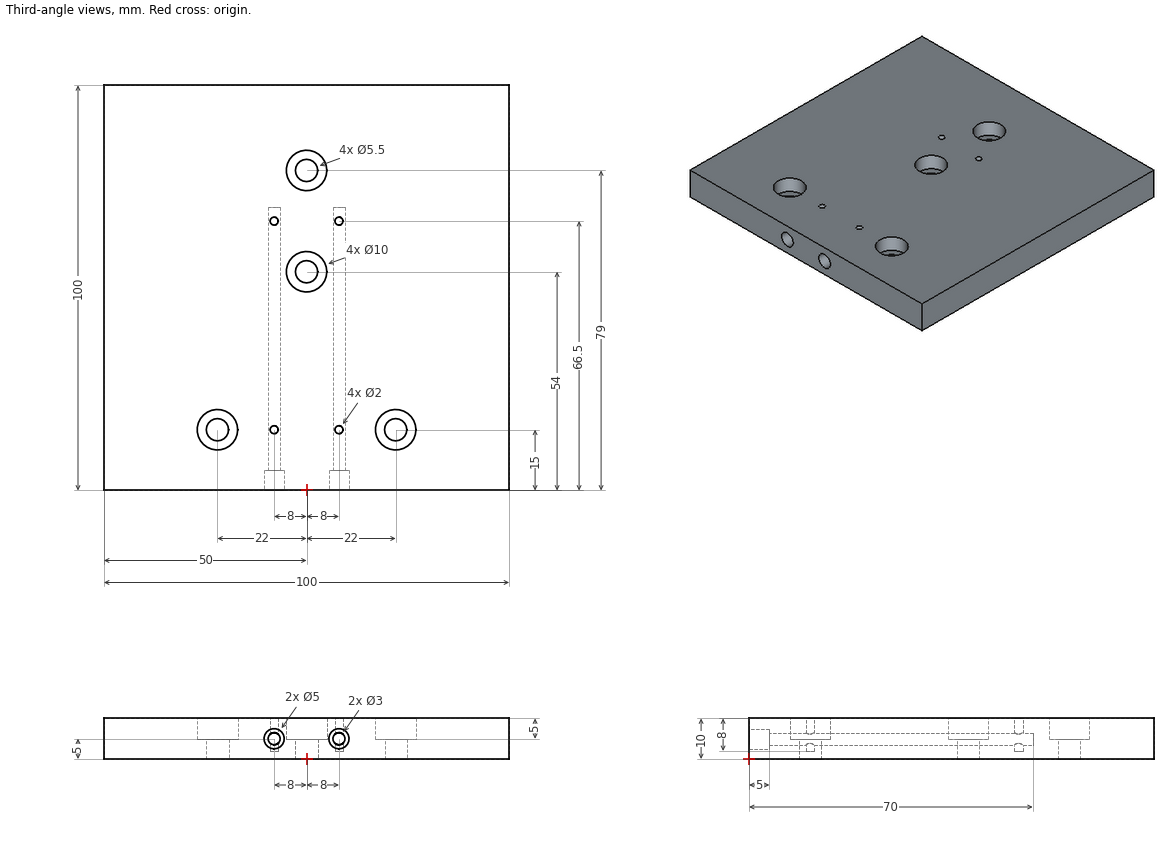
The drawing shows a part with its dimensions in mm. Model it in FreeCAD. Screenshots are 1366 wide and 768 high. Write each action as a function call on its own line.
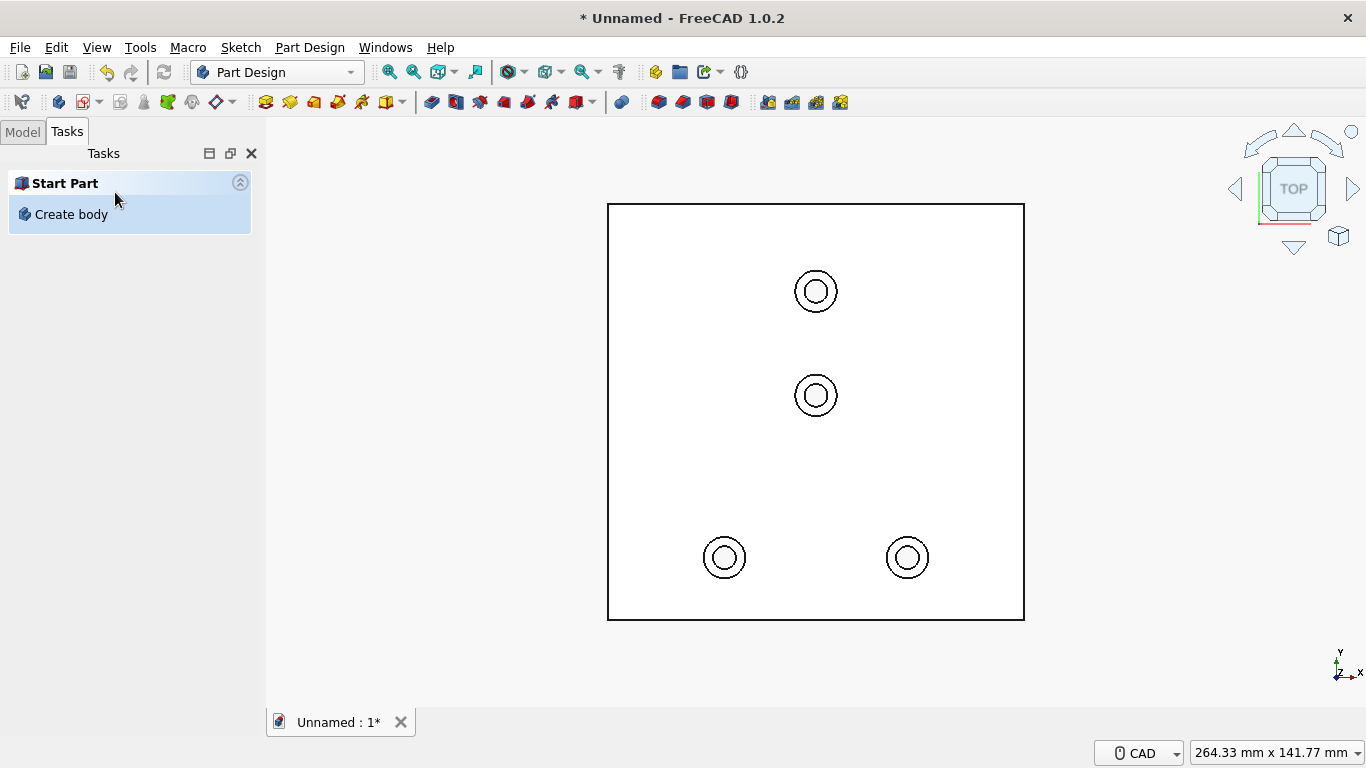
click(935, 352)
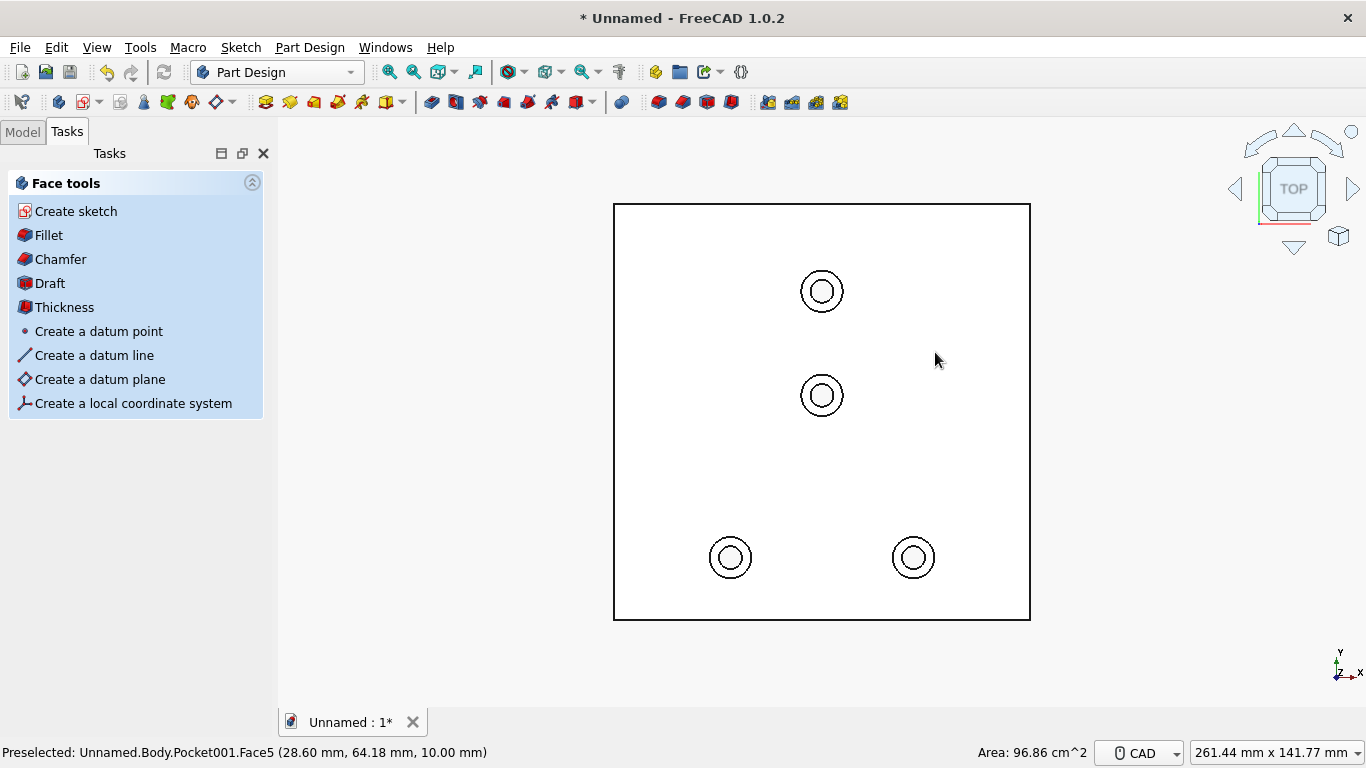
click(84, 102)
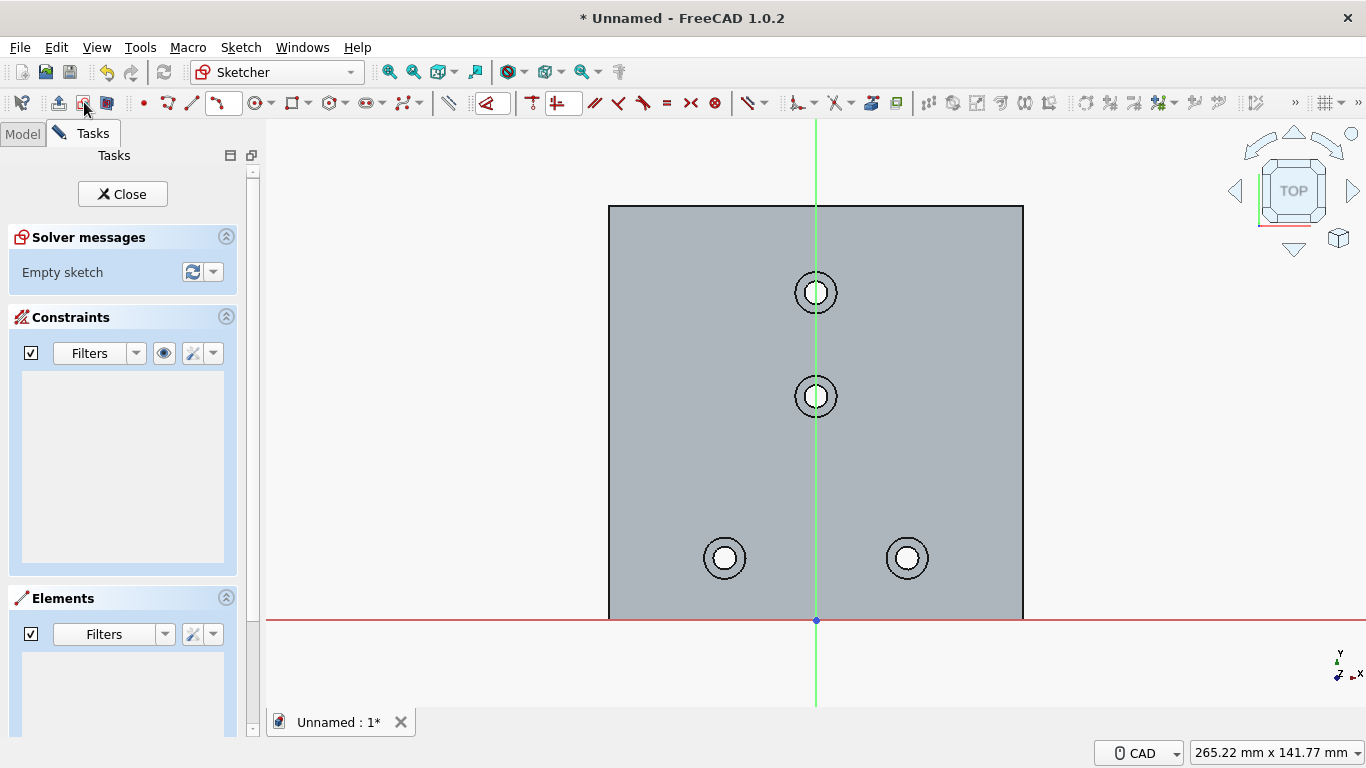
click(256, 104)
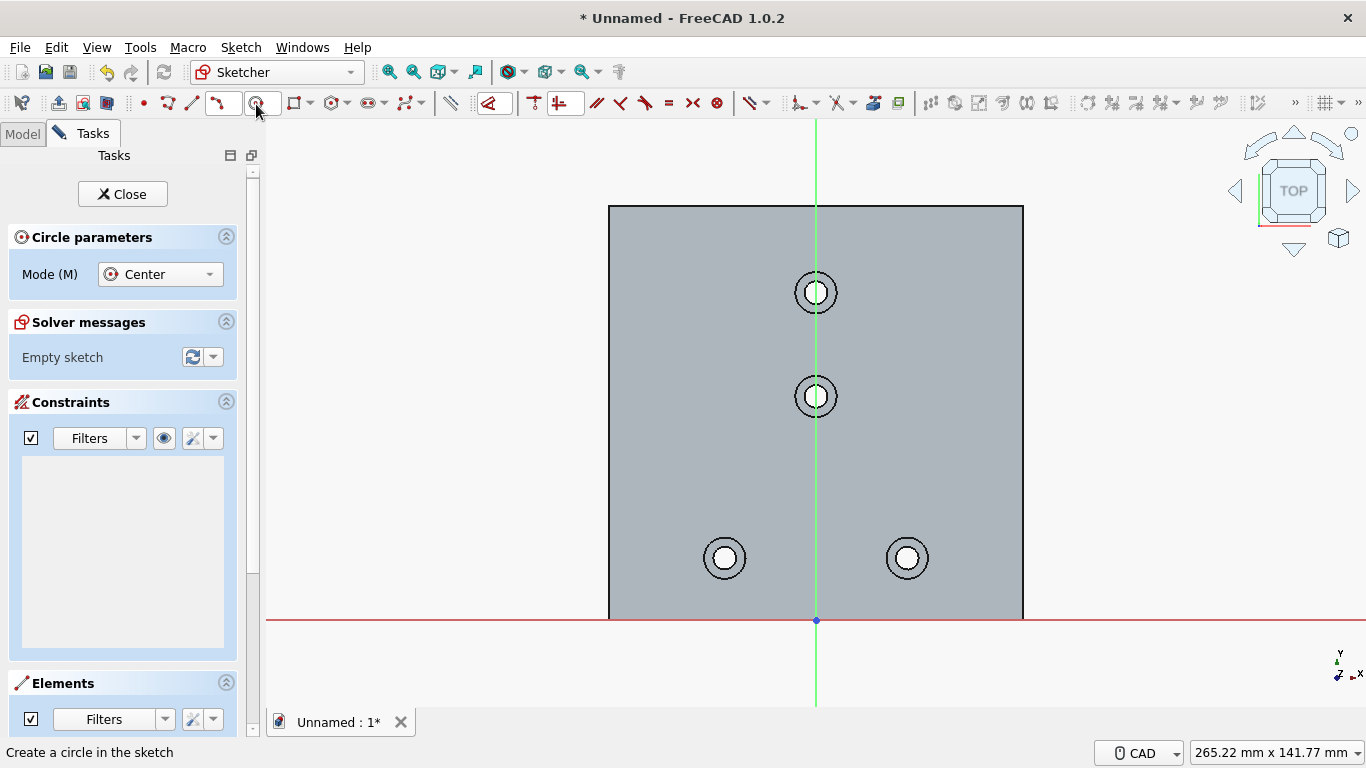
scroll(849, 558, up, 9)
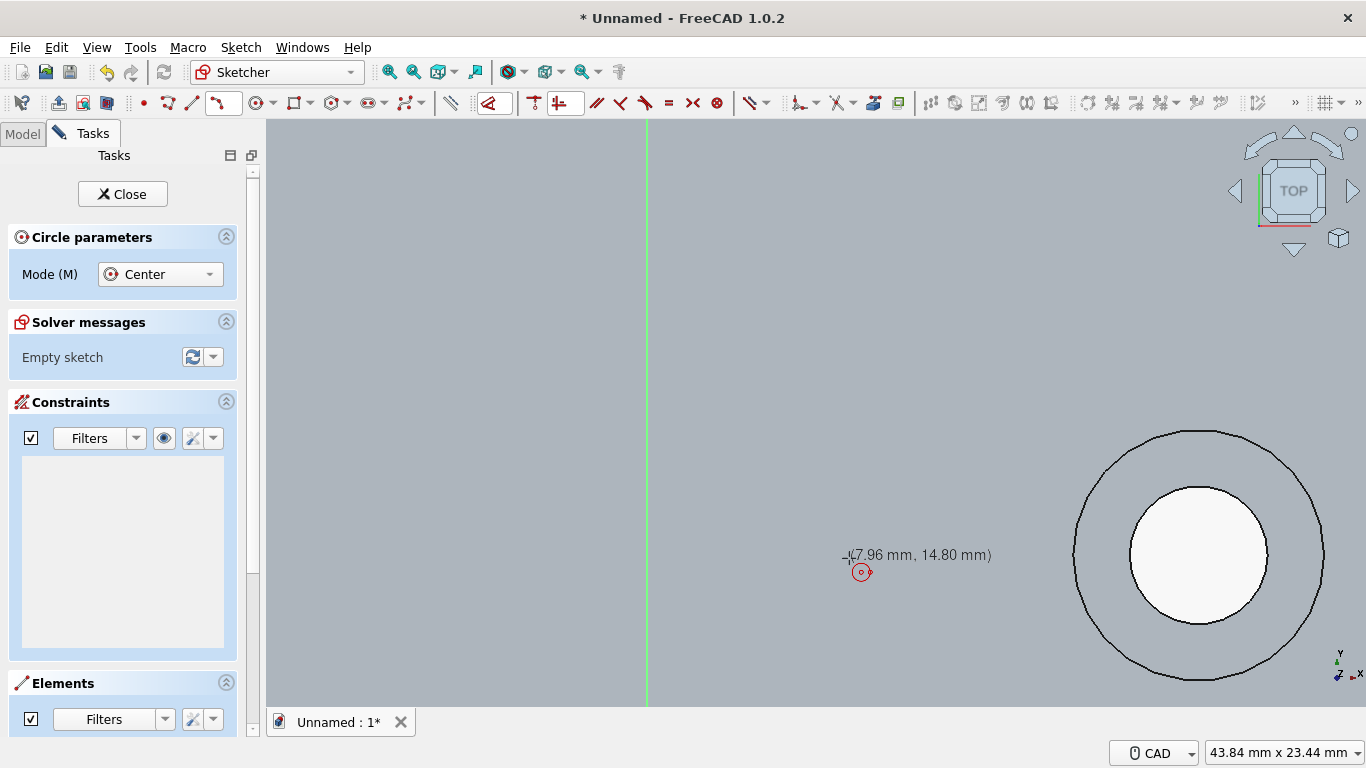
scroll(773, 496, down, 8)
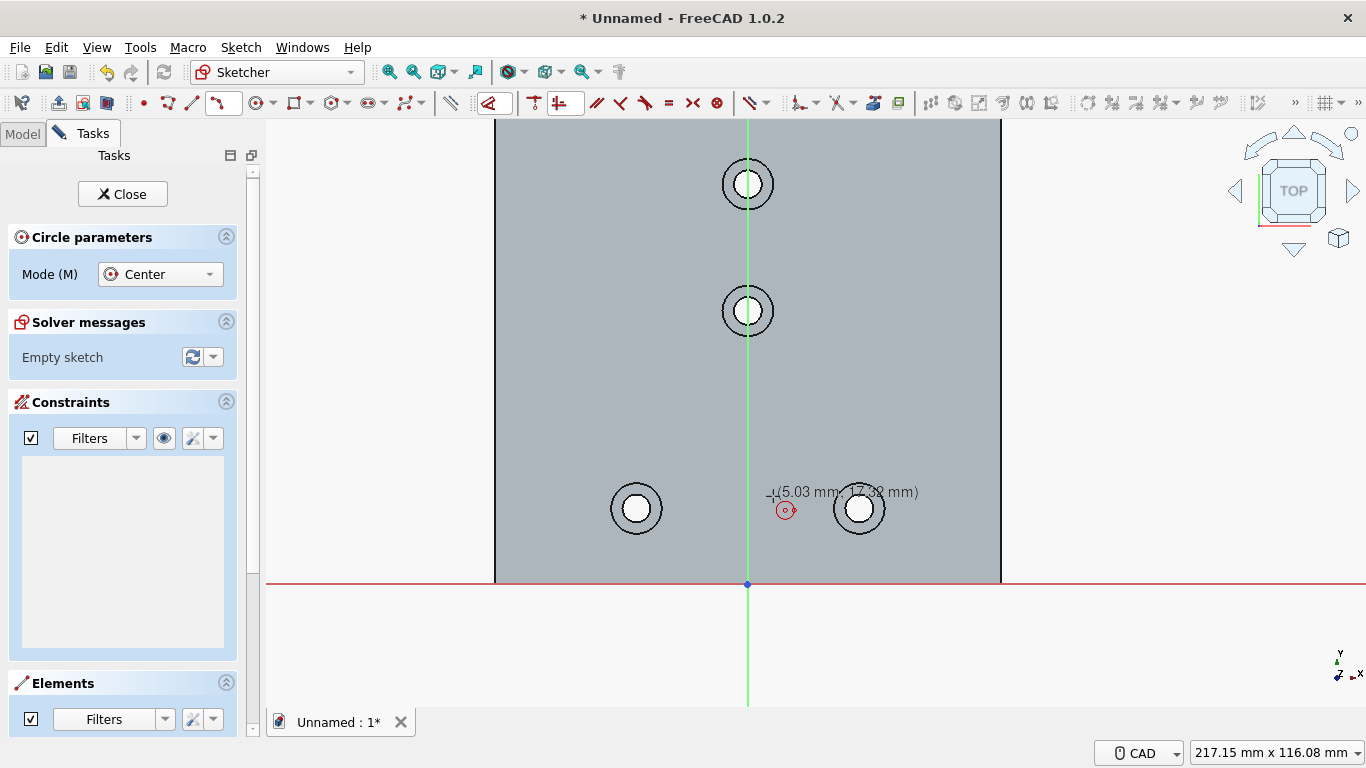
click(788, 508)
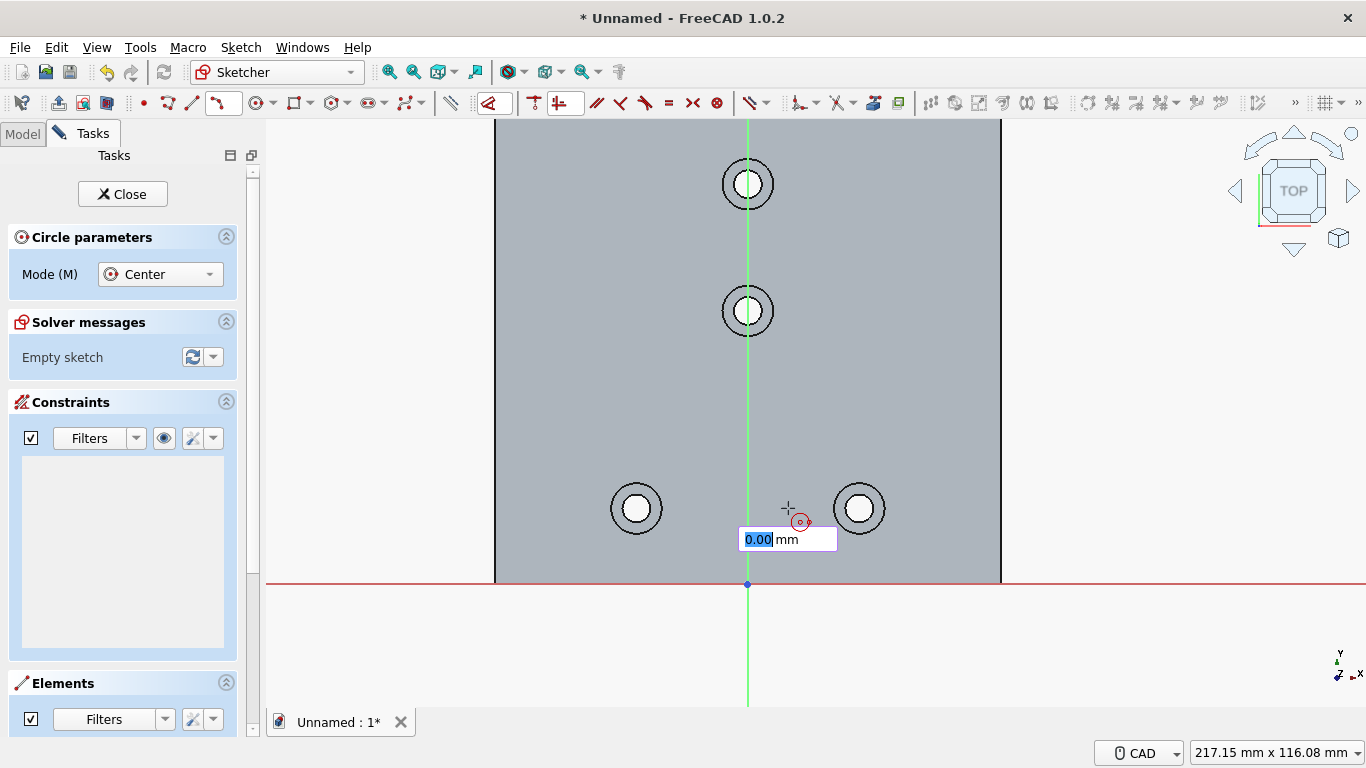
scroll(792, 505, up, 6)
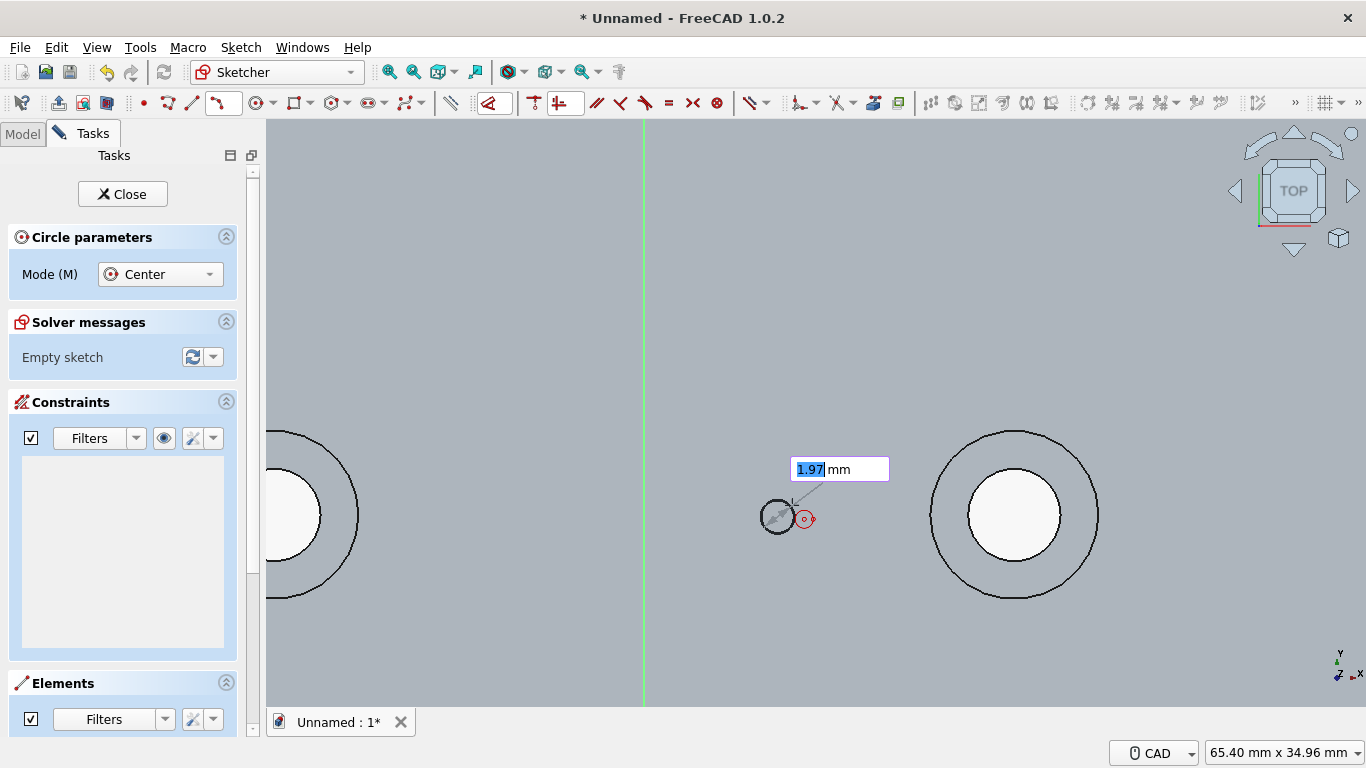
click(791, 503)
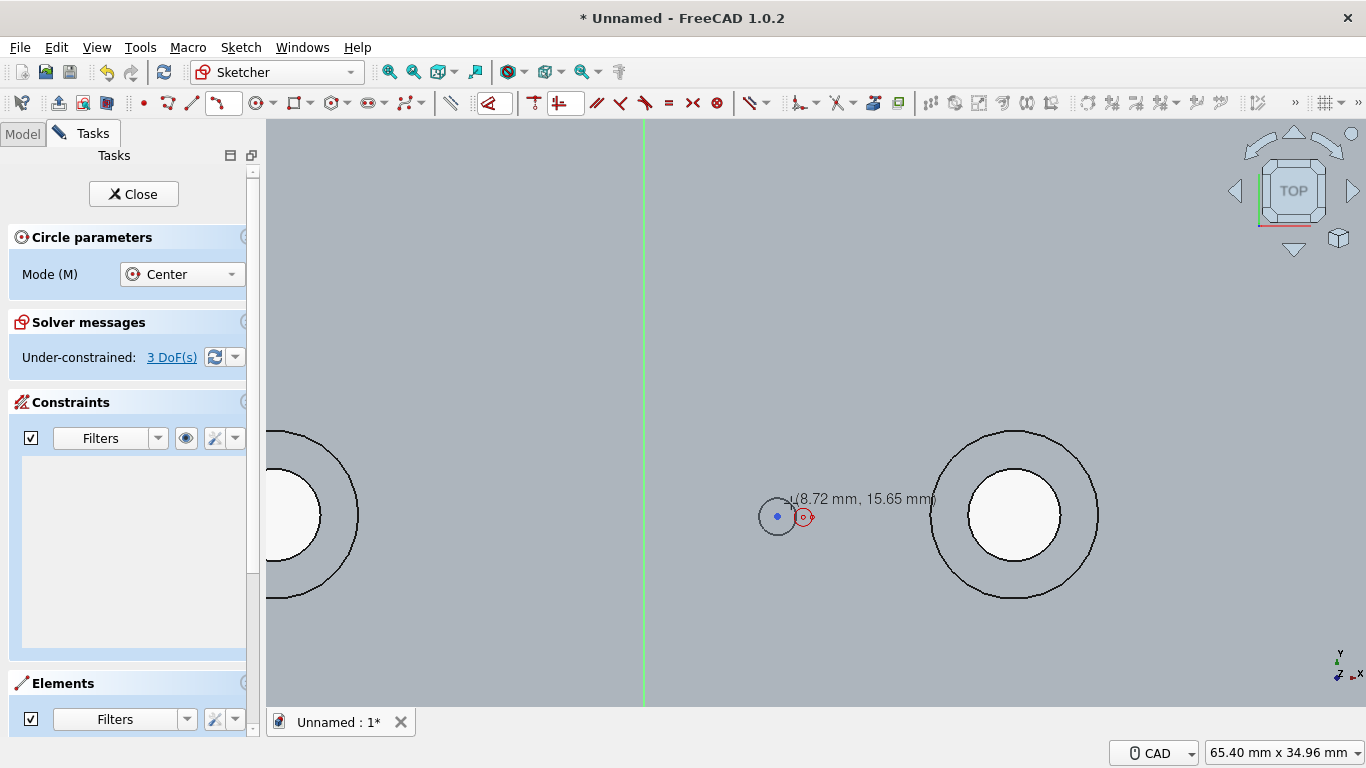
scroll(510, 515, up, 2)